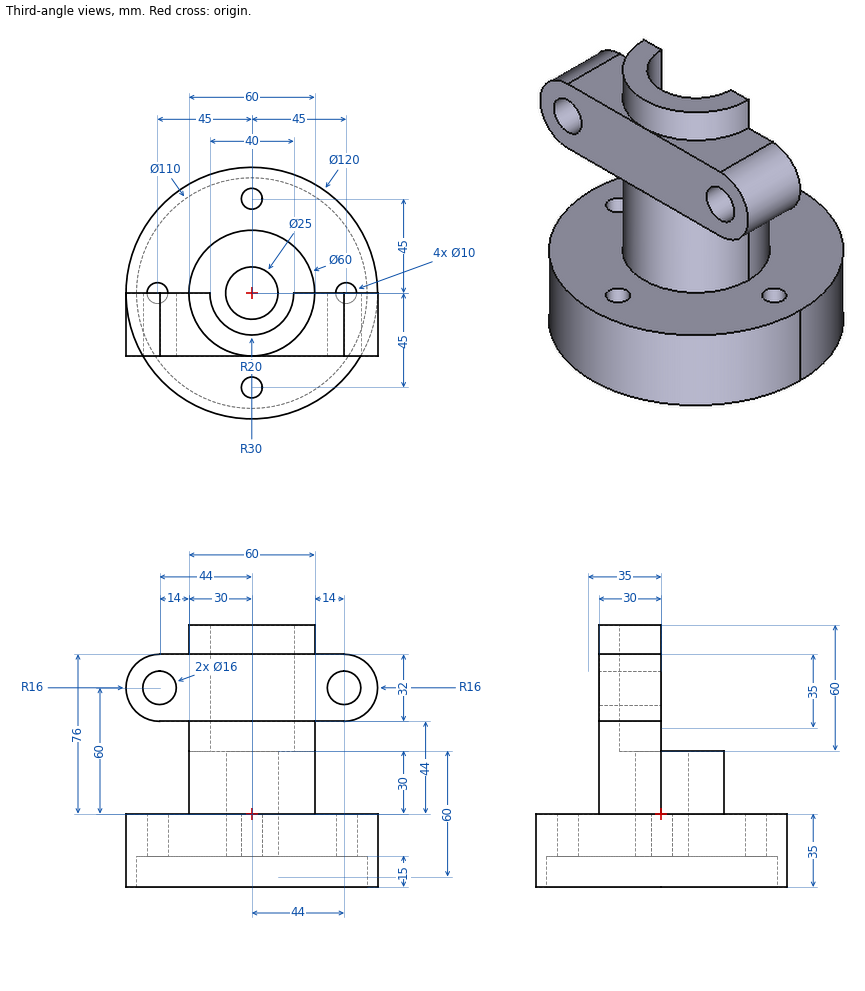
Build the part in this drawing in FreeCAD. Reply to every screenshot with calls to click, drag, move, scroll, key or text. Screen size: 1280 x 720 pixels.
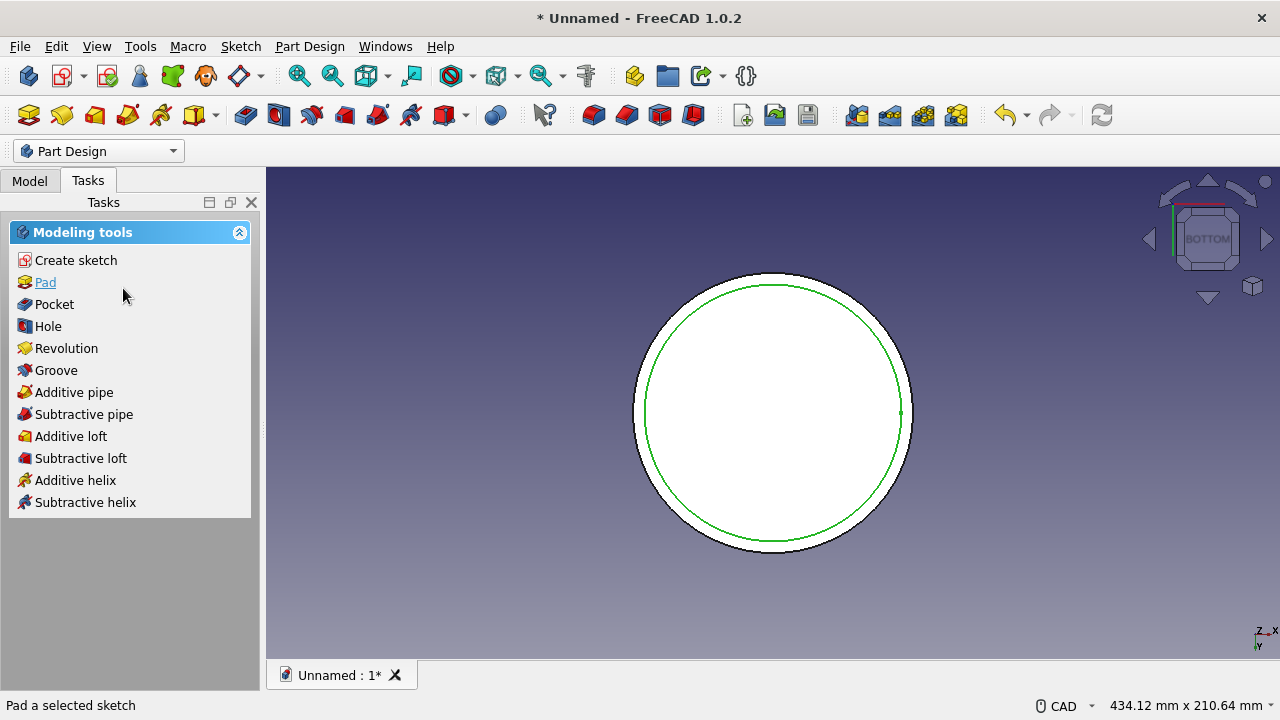
click(246, 116)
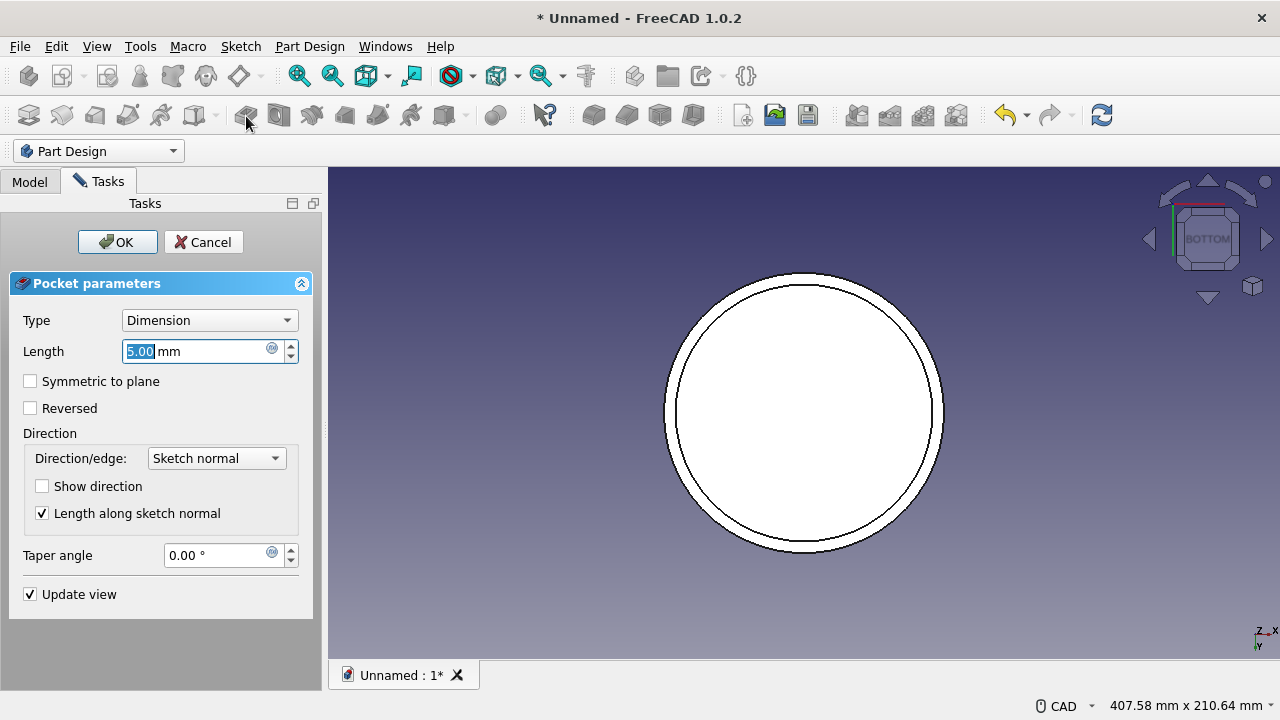
text(15)
key(Tab)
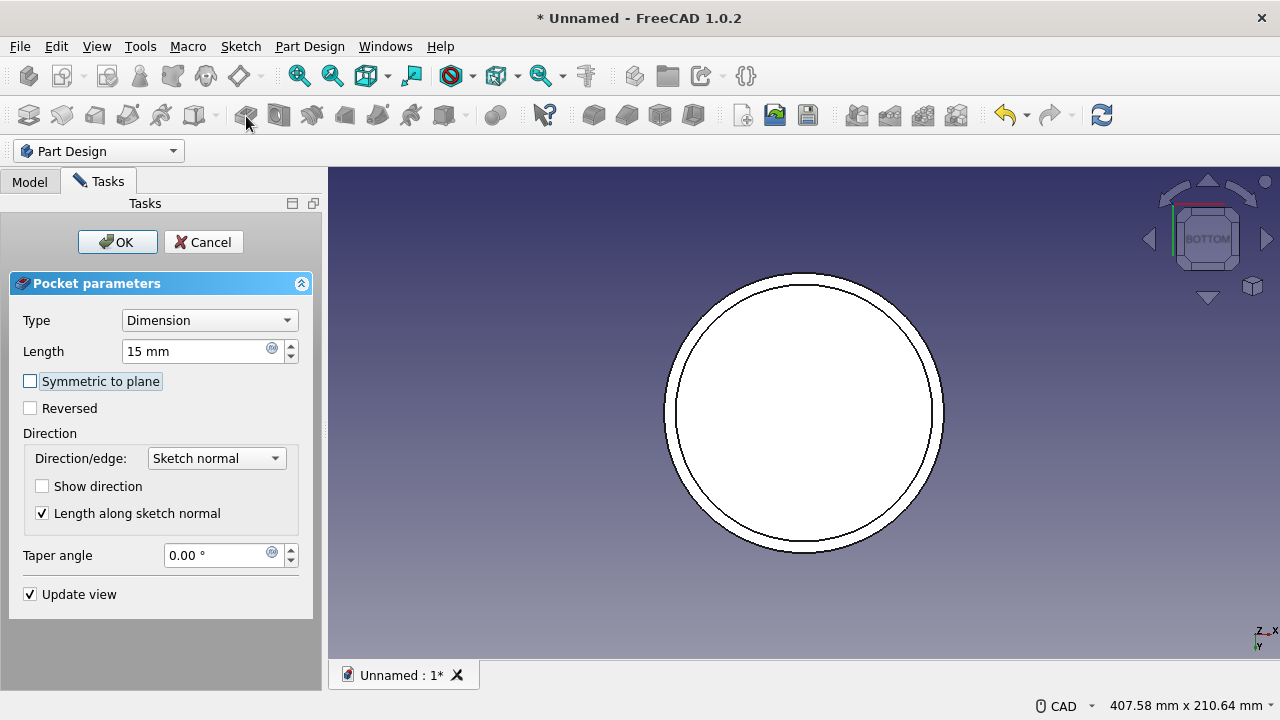
click(118, 242)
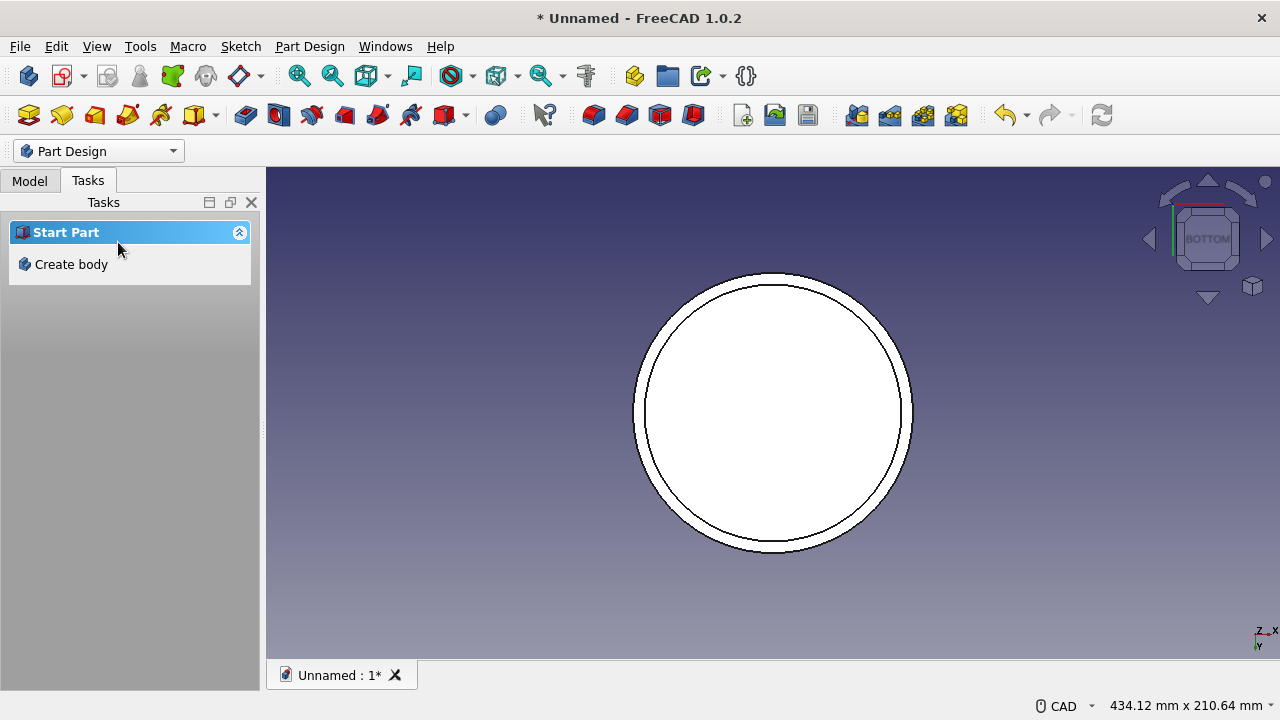
key(0)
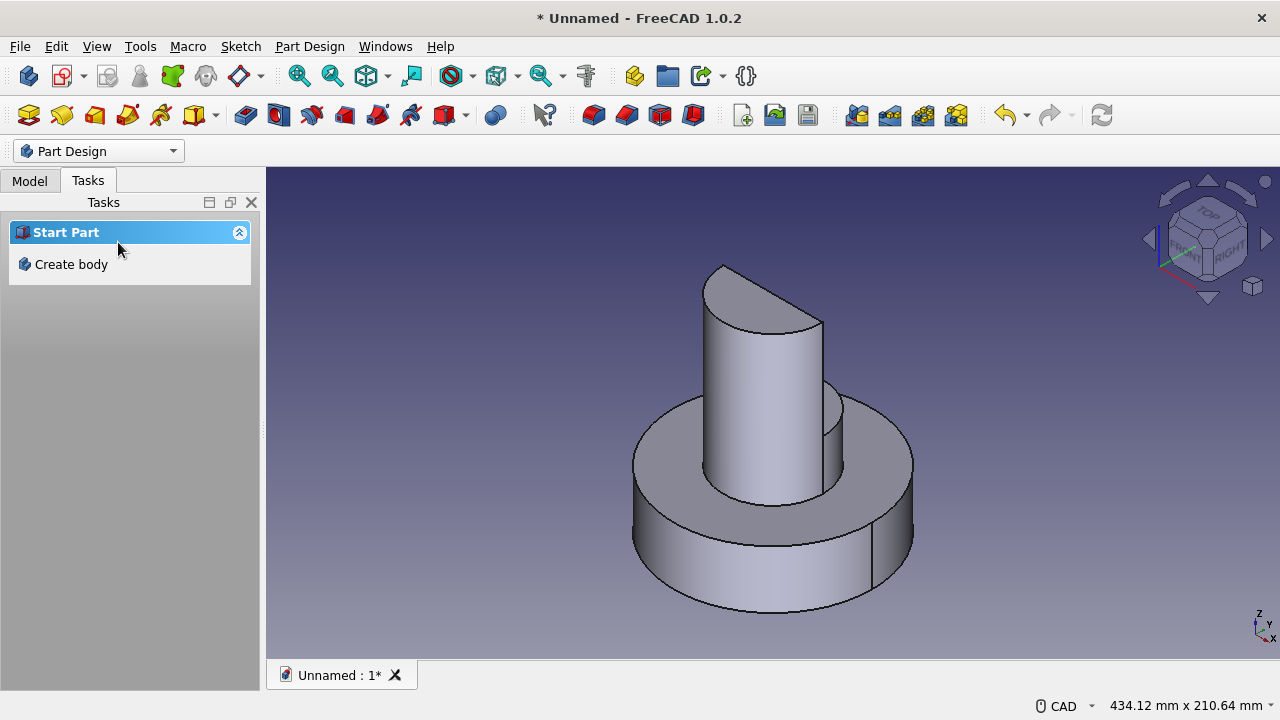
click(660, 464)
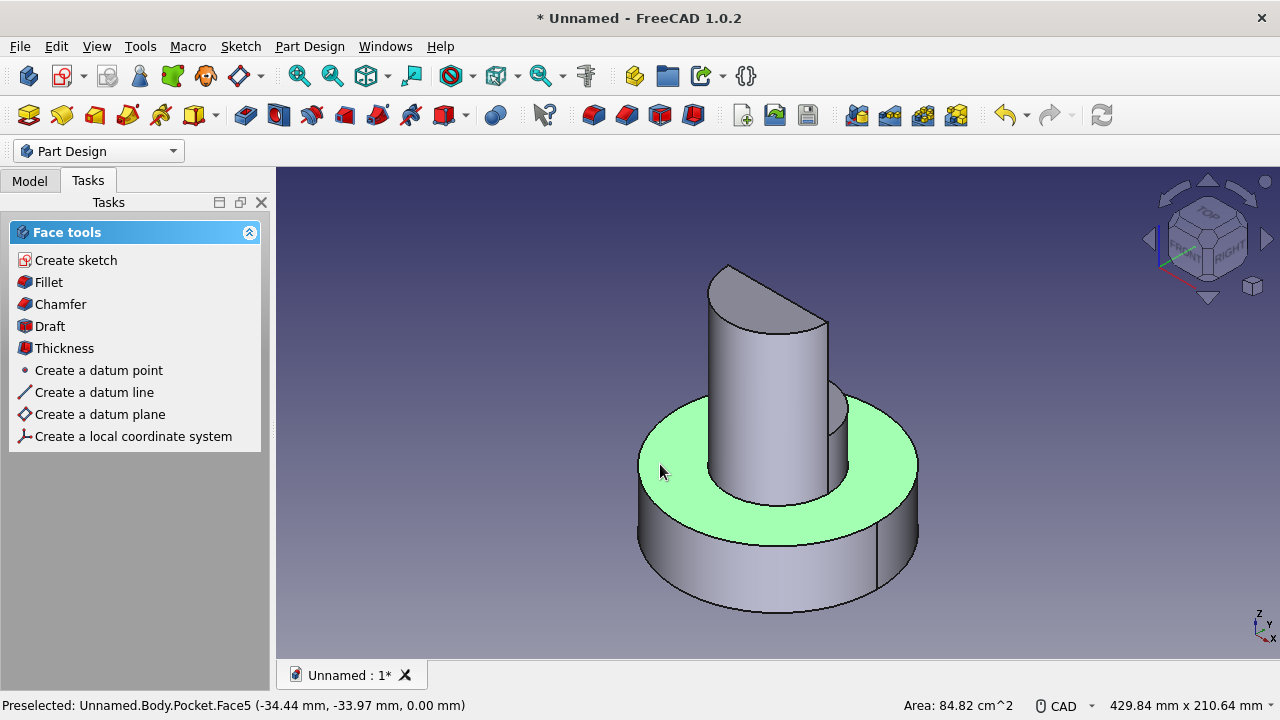
click(62, 76)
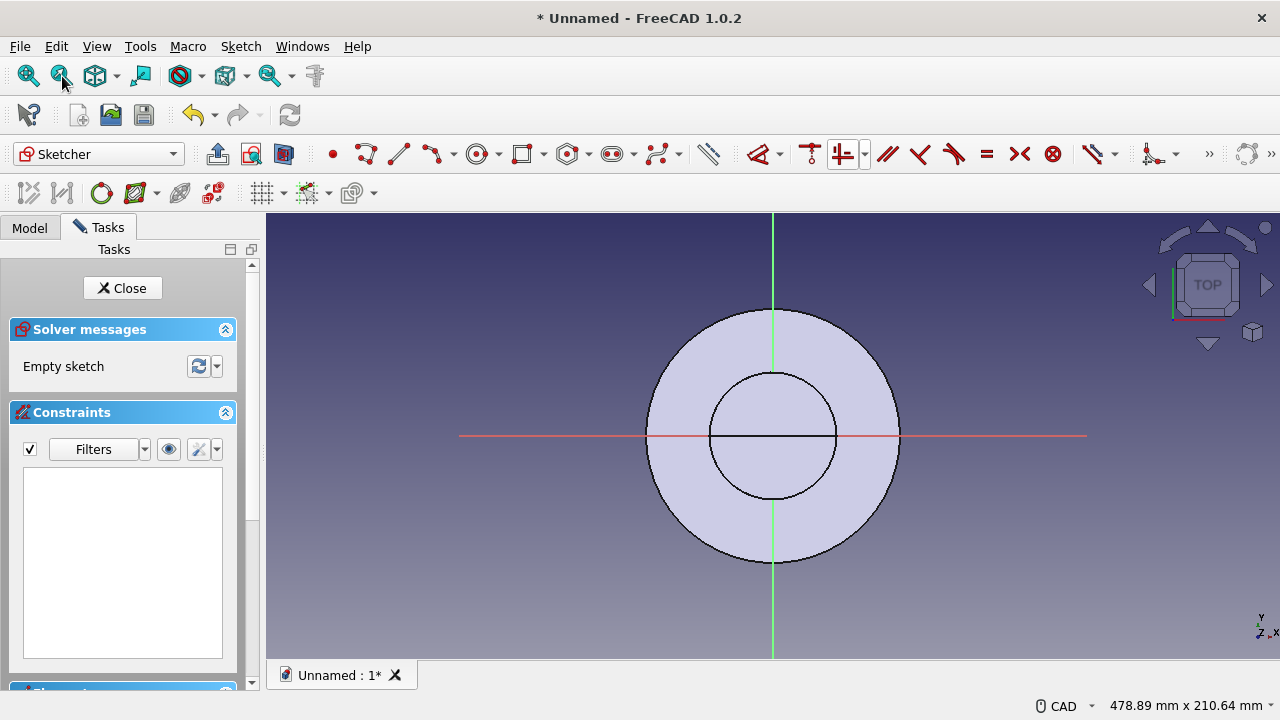
click(284, 154)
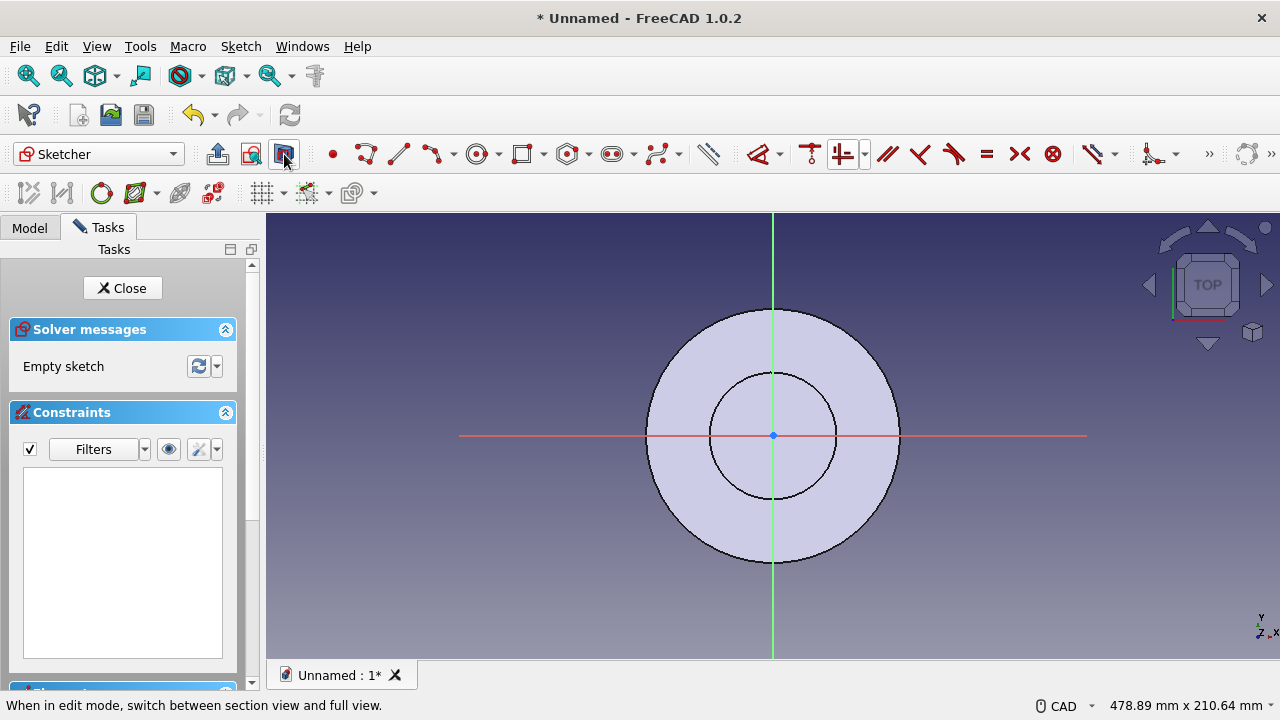
click(476, 154)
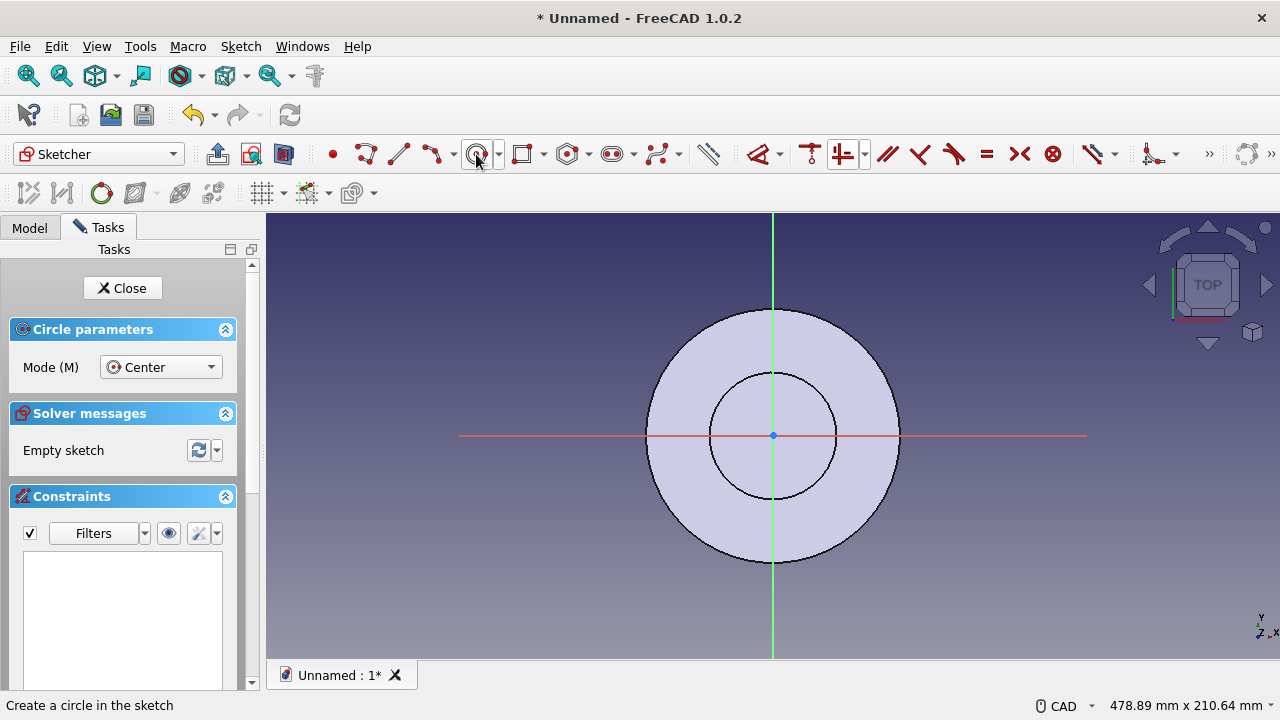
scroll(868, 436, up, 4)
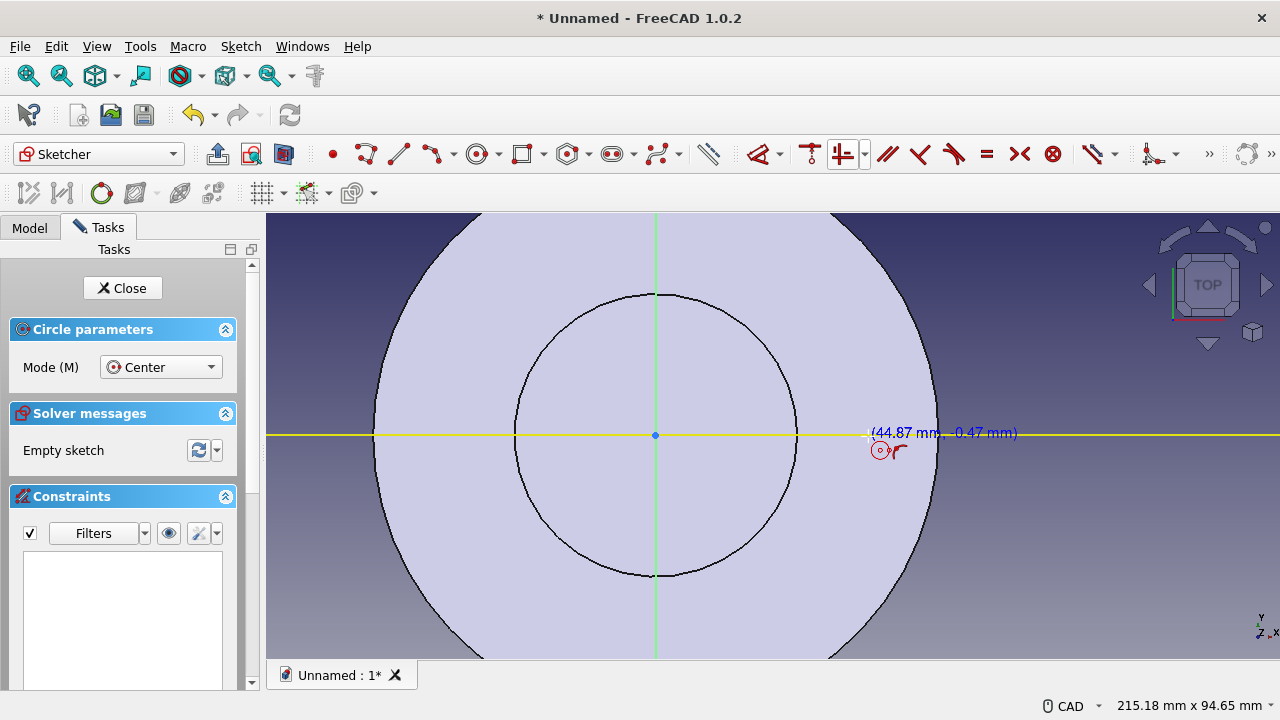
click(868, 435)
move(885, 419)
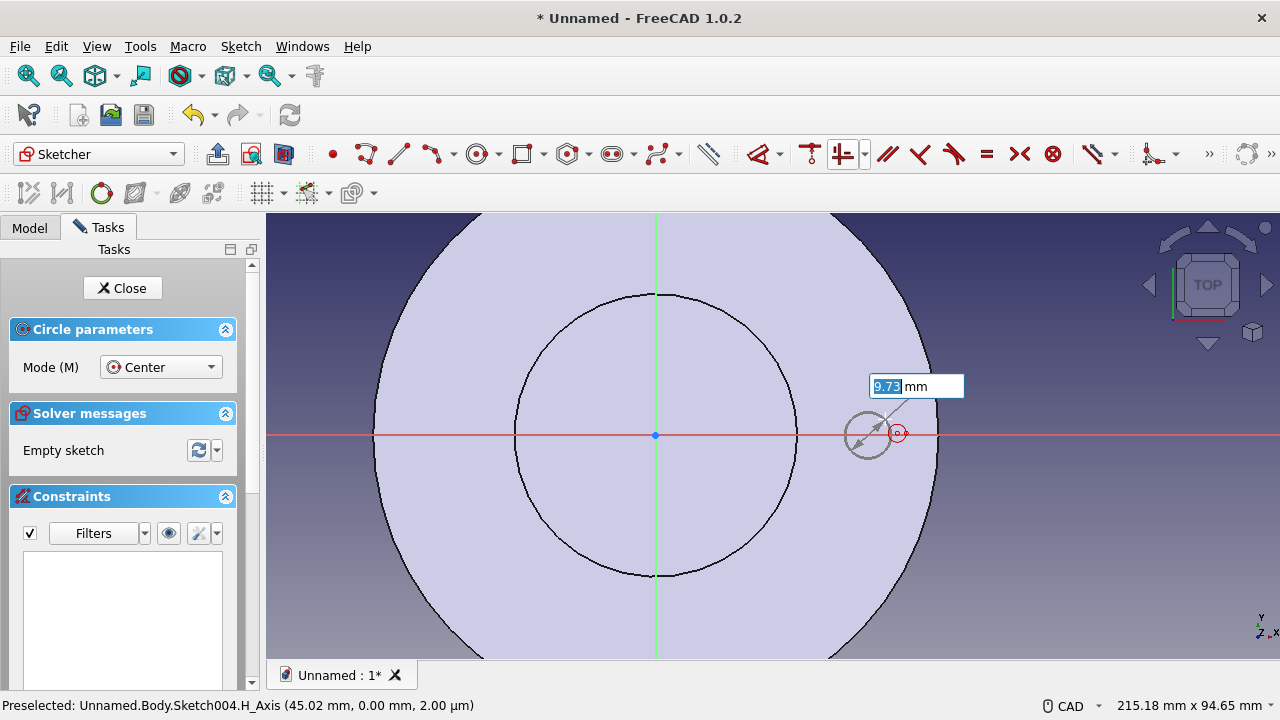
text(10)
key(Return)